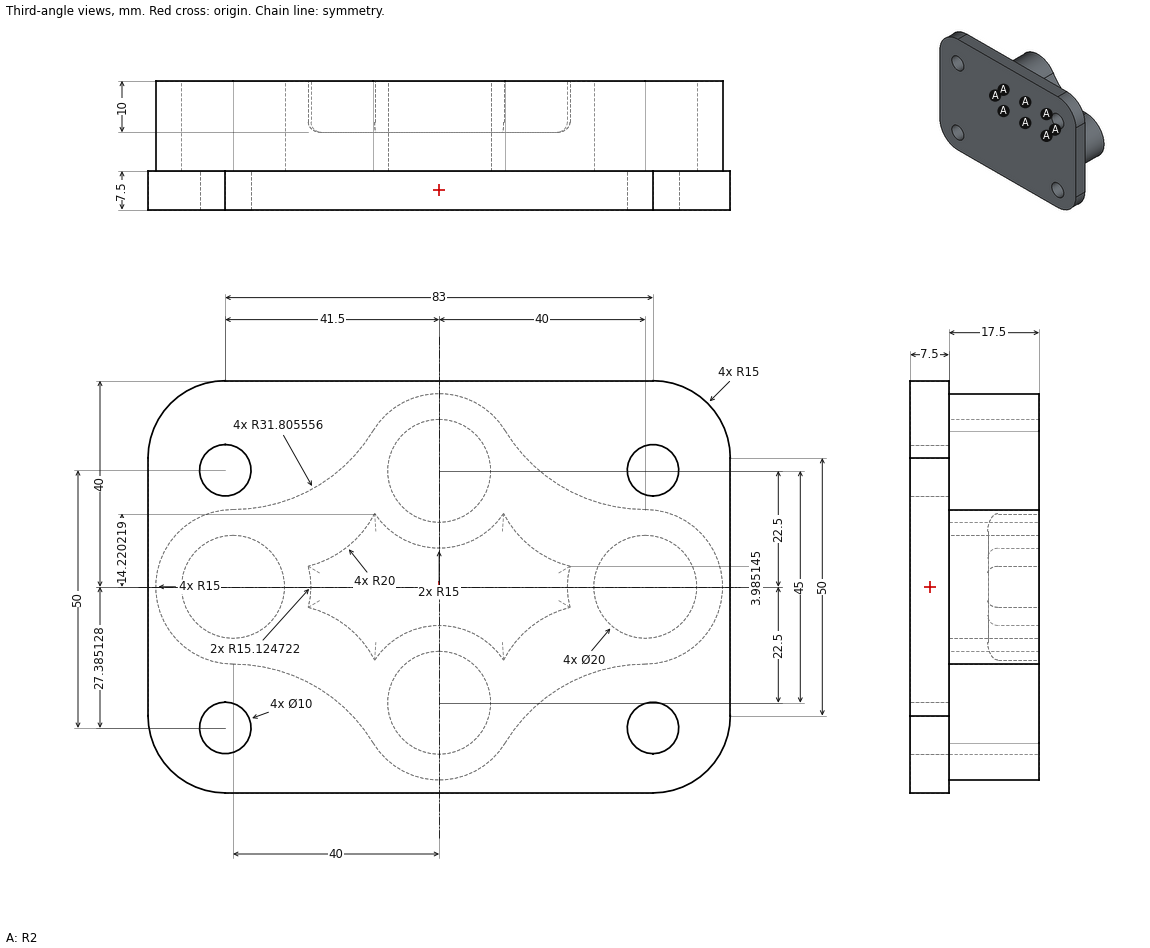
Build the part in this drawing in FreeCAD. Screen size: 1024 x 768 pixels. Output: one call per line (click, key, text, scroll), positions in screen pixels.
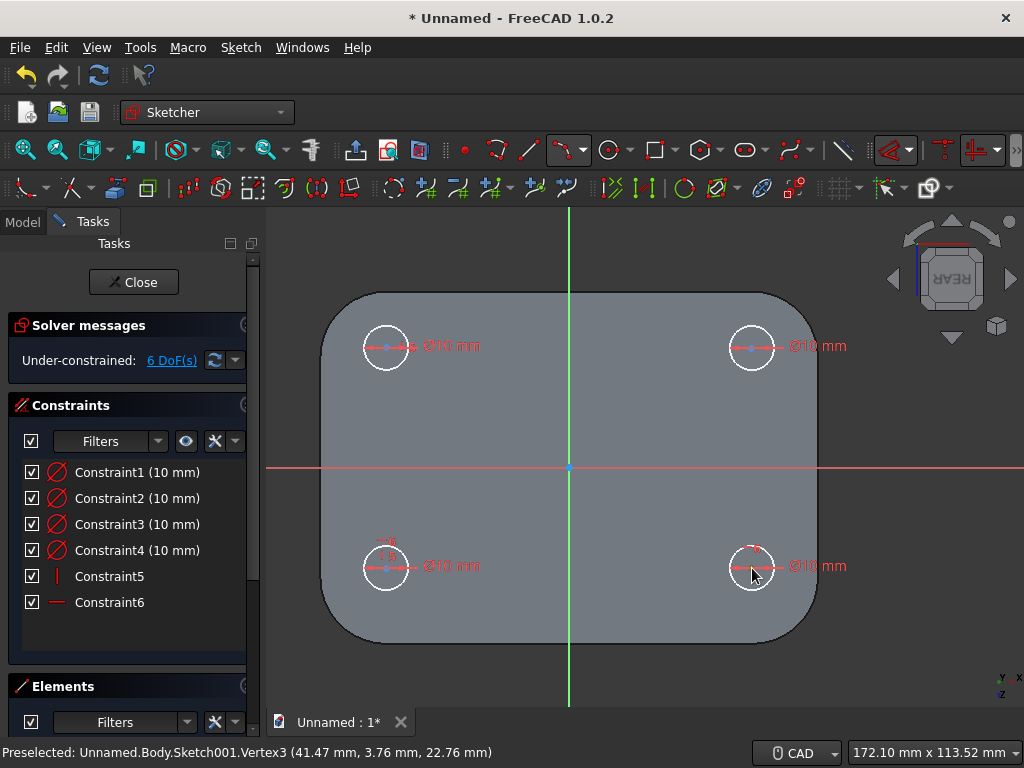
click(752, 348)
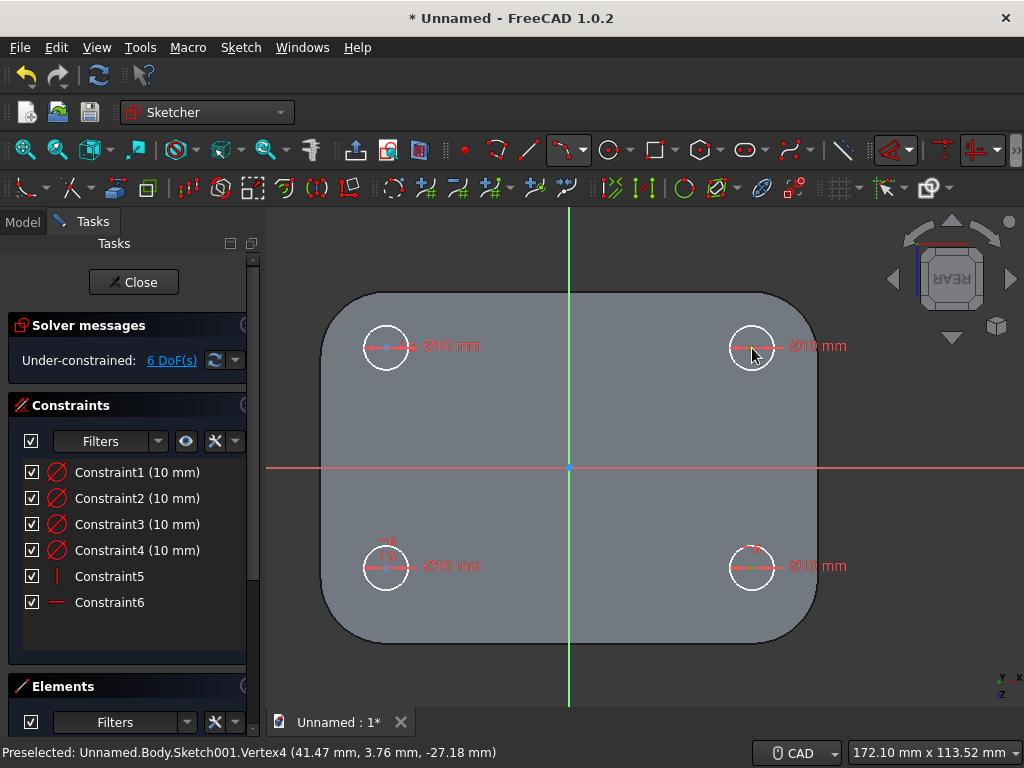
key(v)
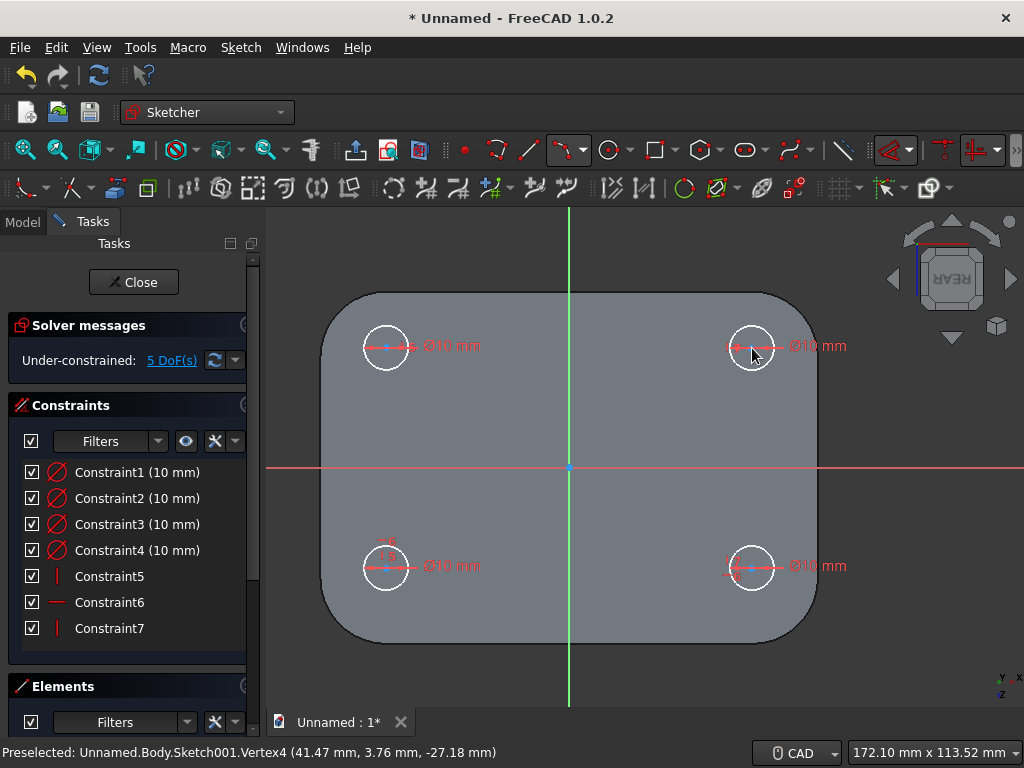
click(386, 348)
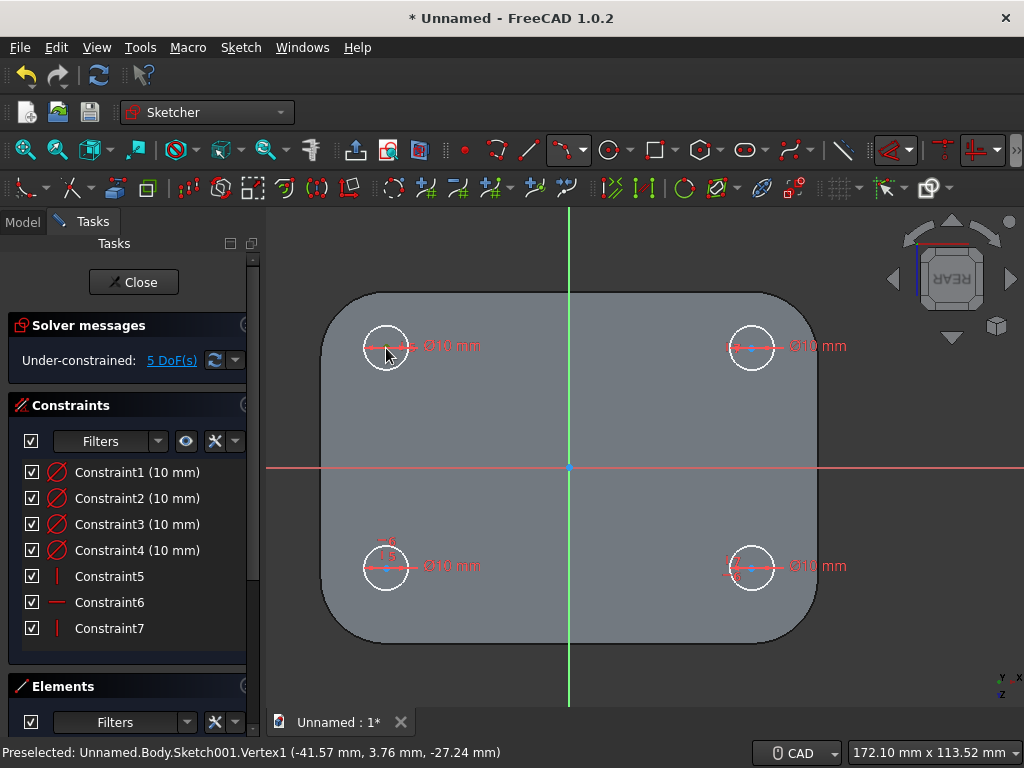
click(752, 348)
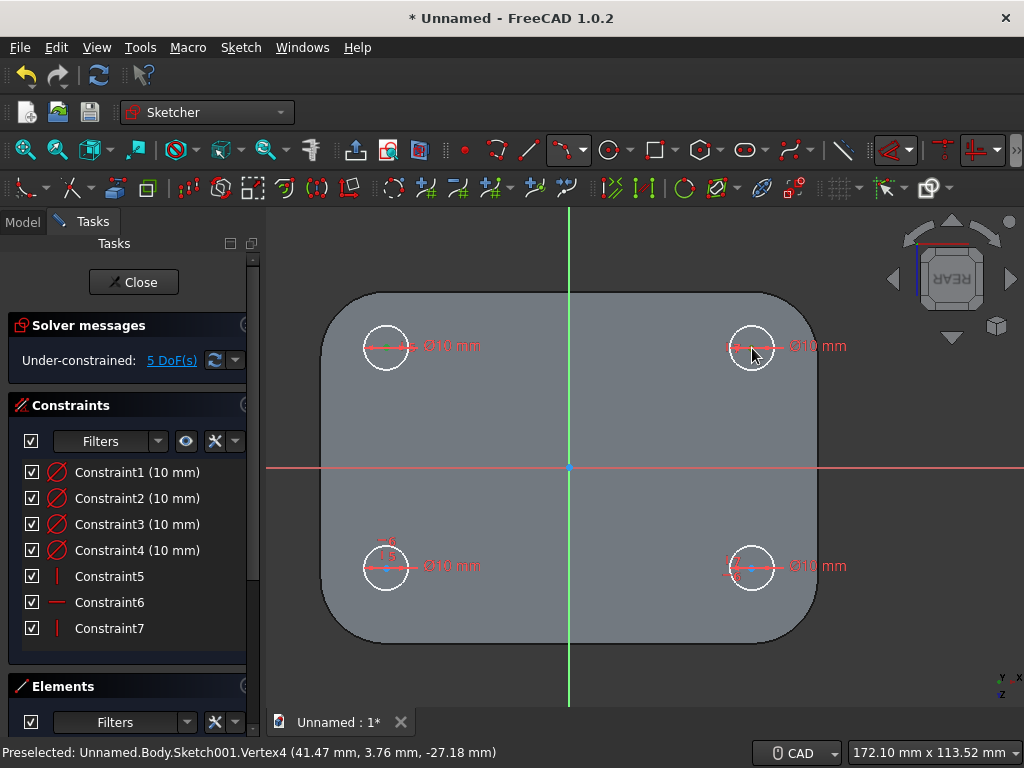
click(1000, 150)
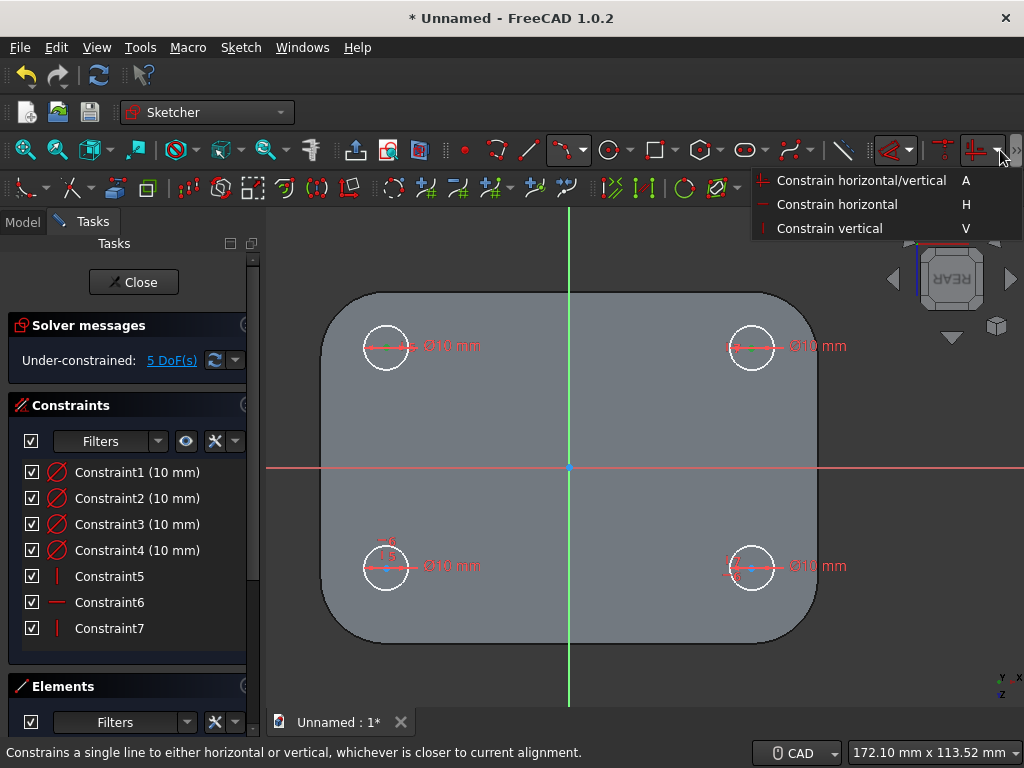
click(887, 204)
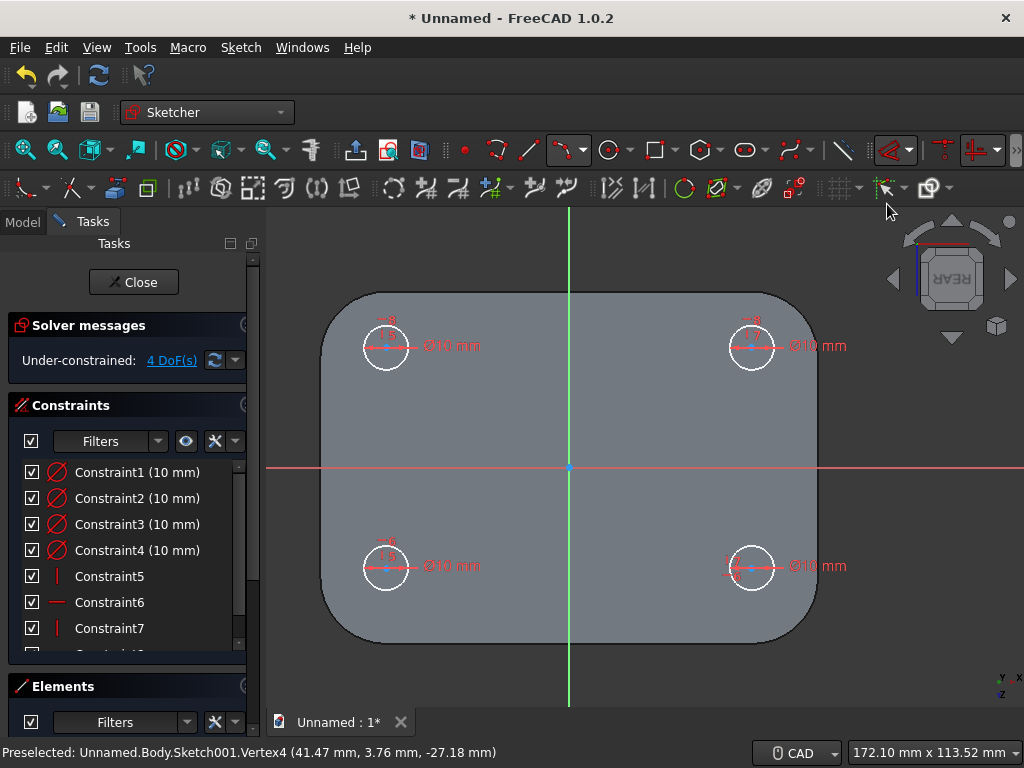
click(386, 348)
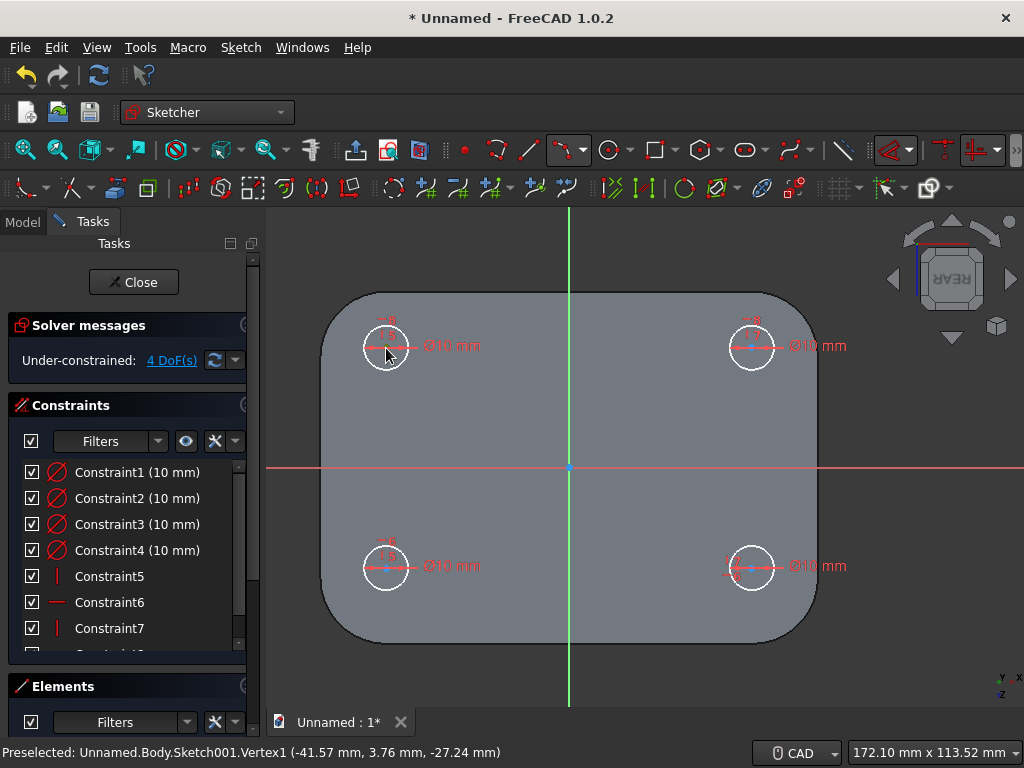
click(386, 568)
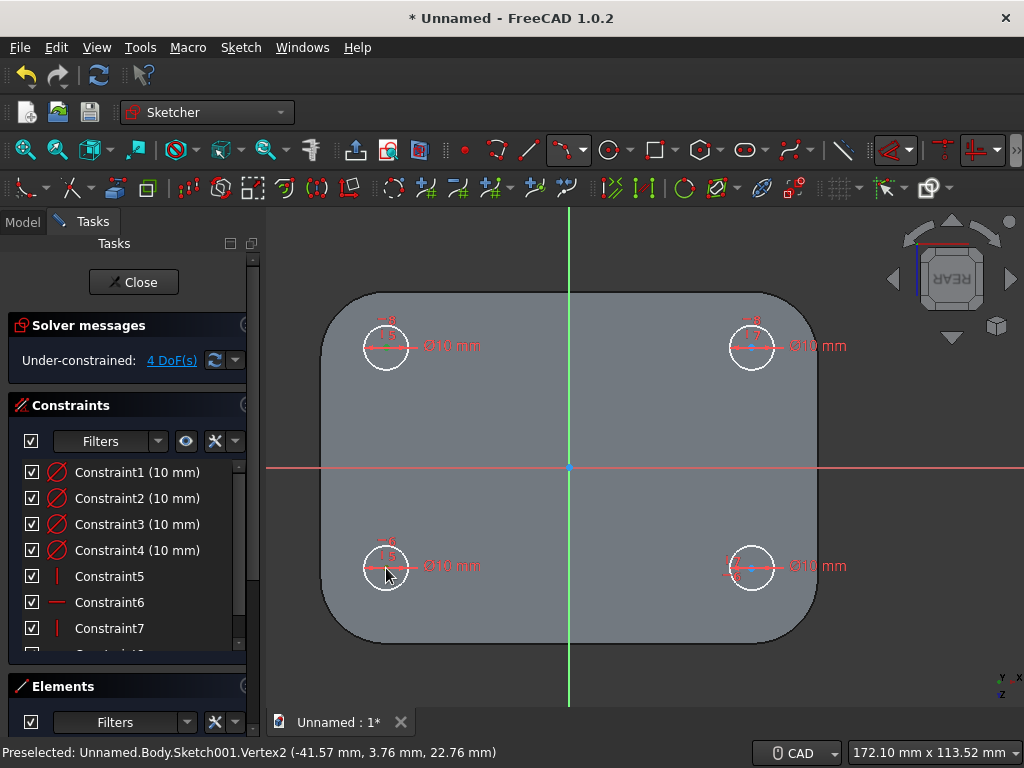
click(912, 150)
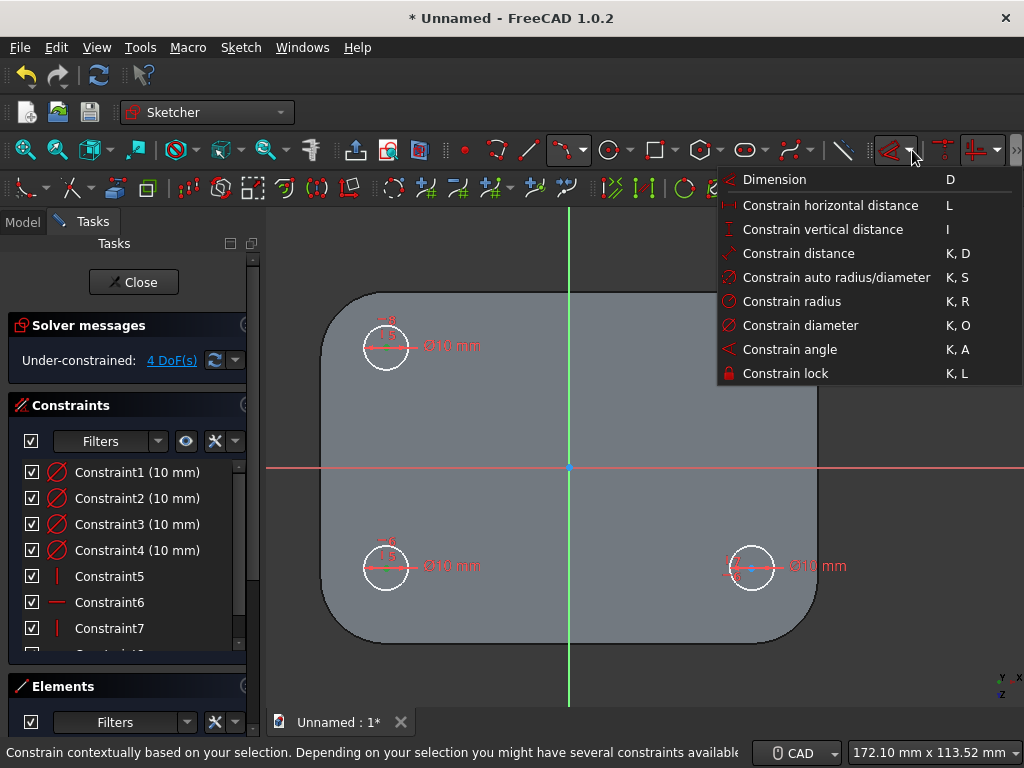
click(870, 229)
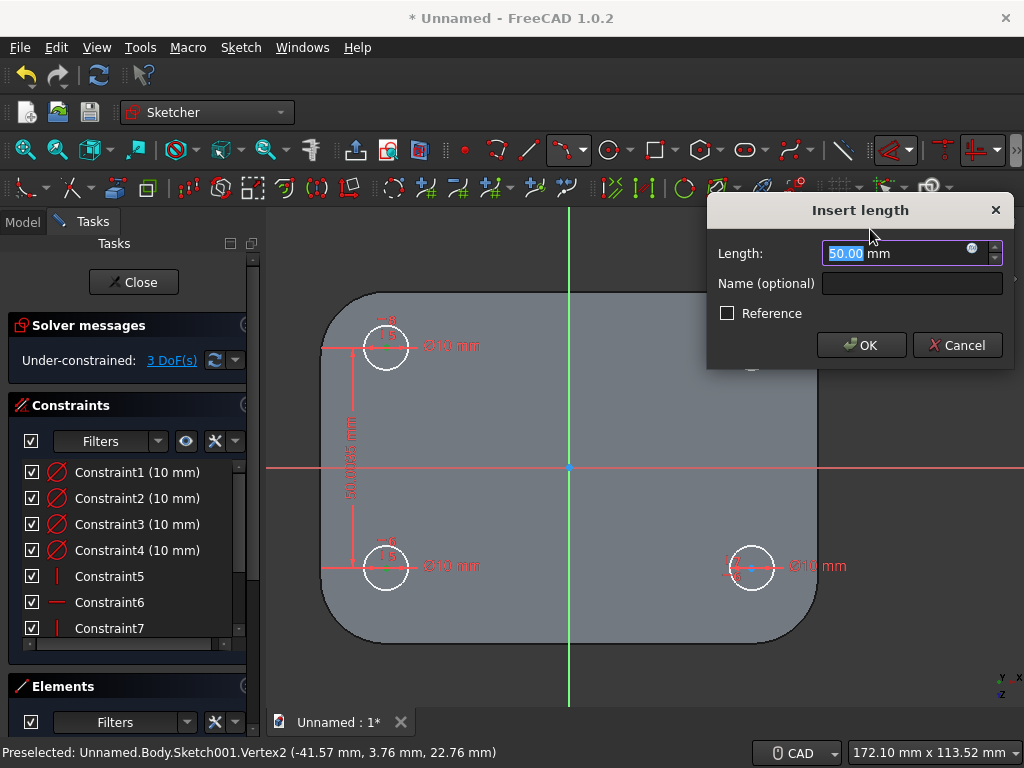
text(50)
key(Return)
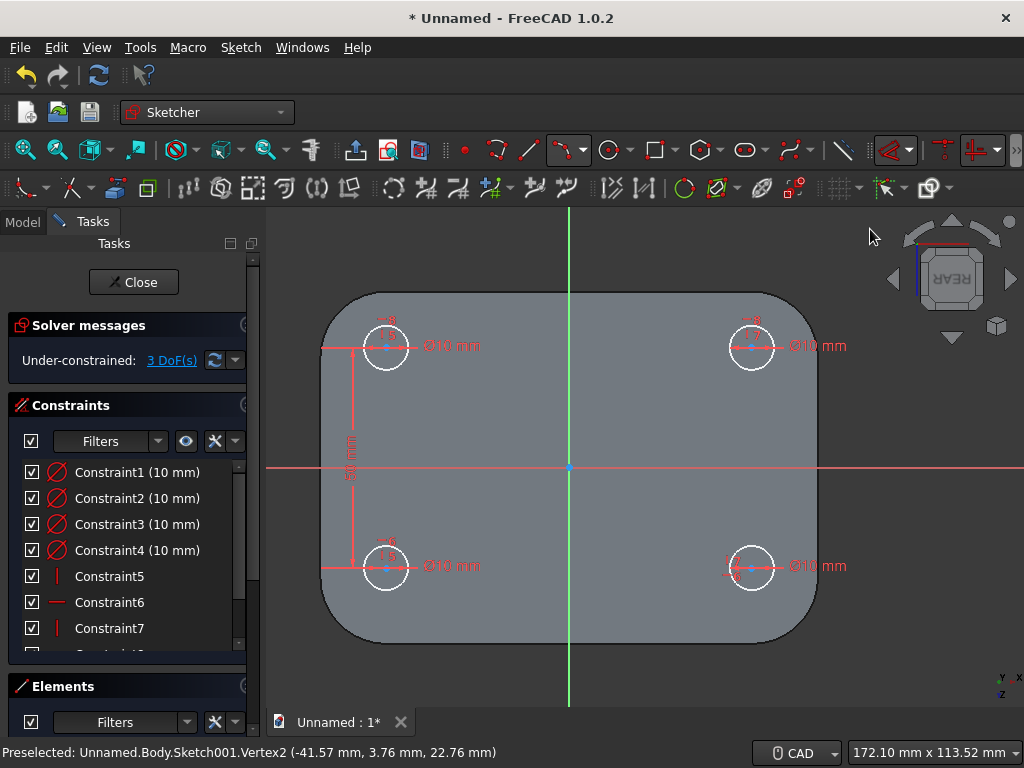
click(386, 568)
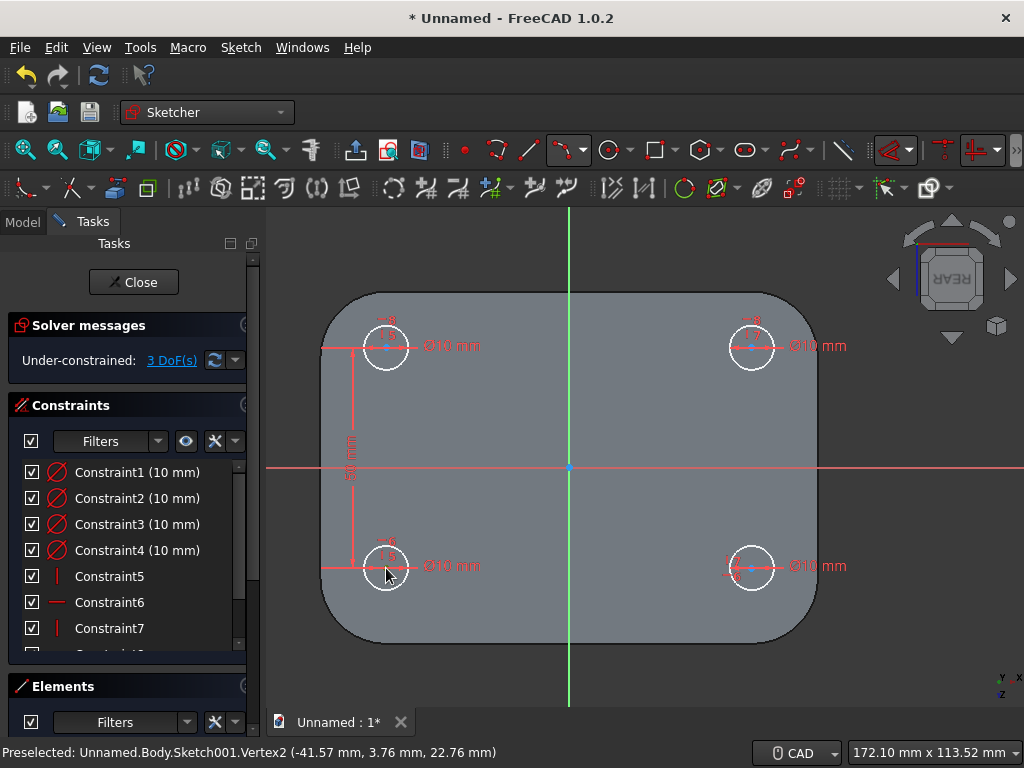
click(752, 568)